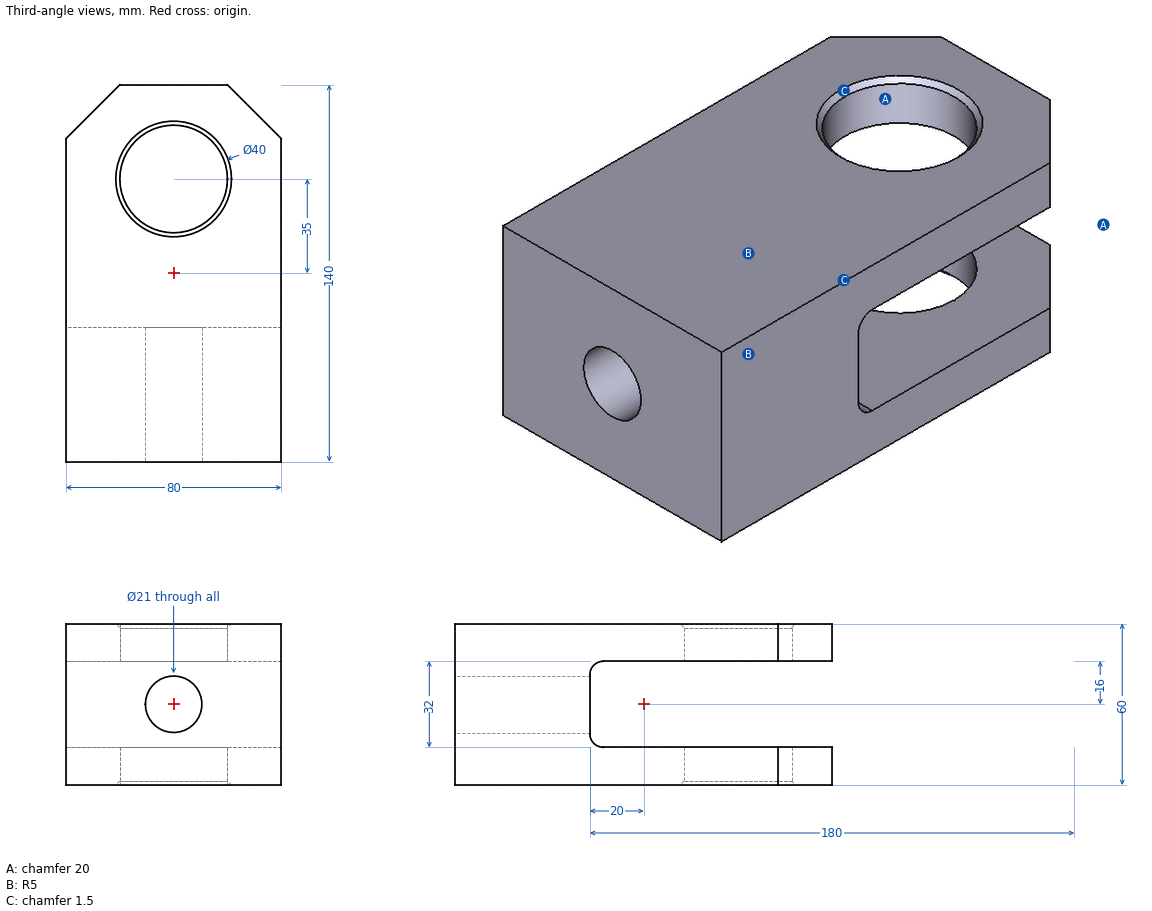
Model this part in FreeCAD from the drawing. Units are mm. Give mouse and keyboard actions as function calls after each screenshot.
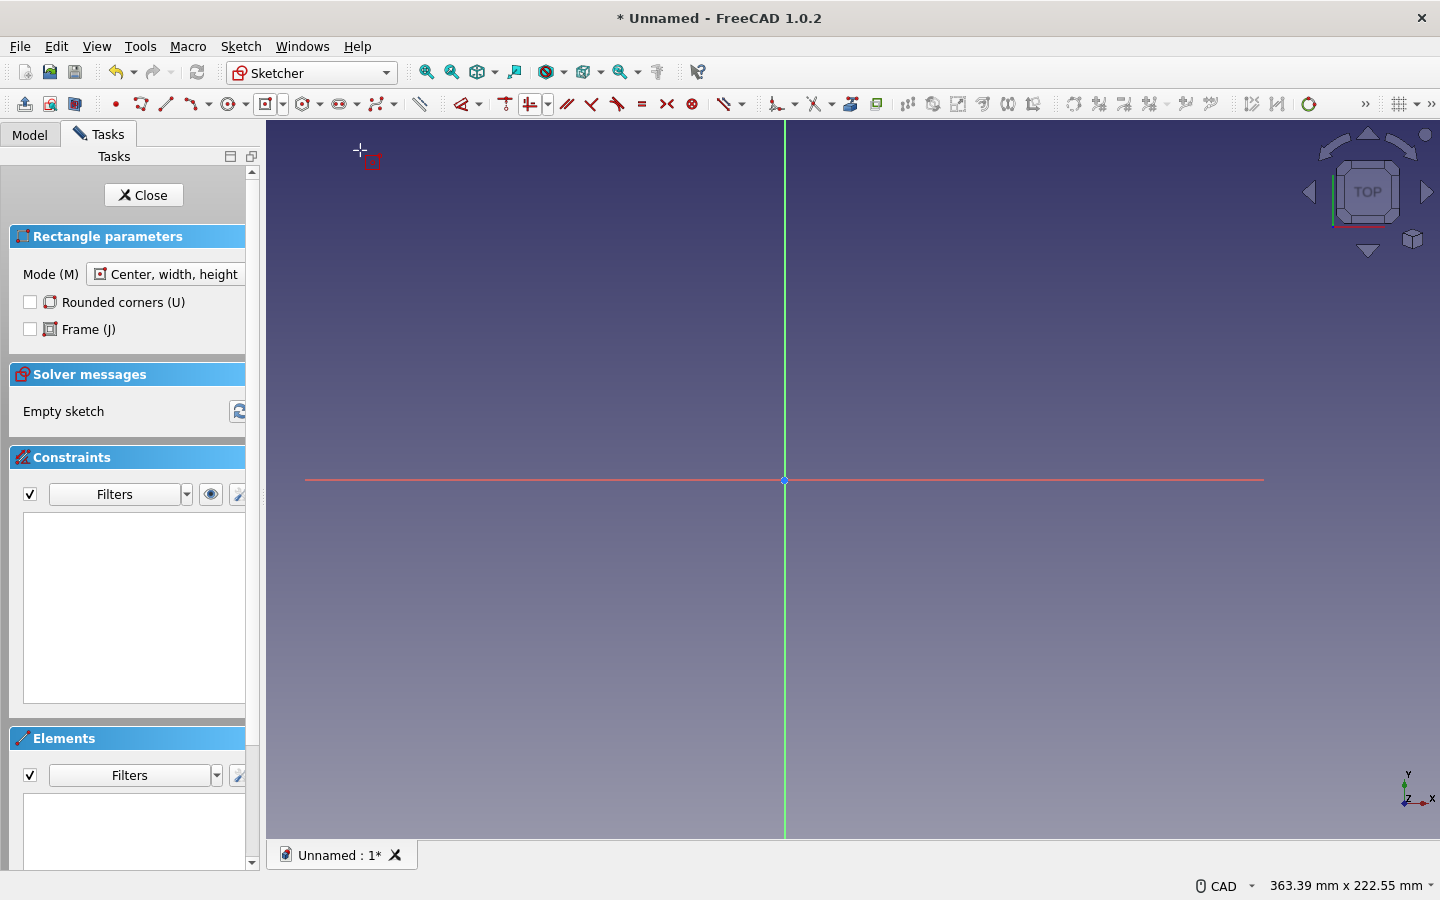
click(785, 480)
move(914, 254)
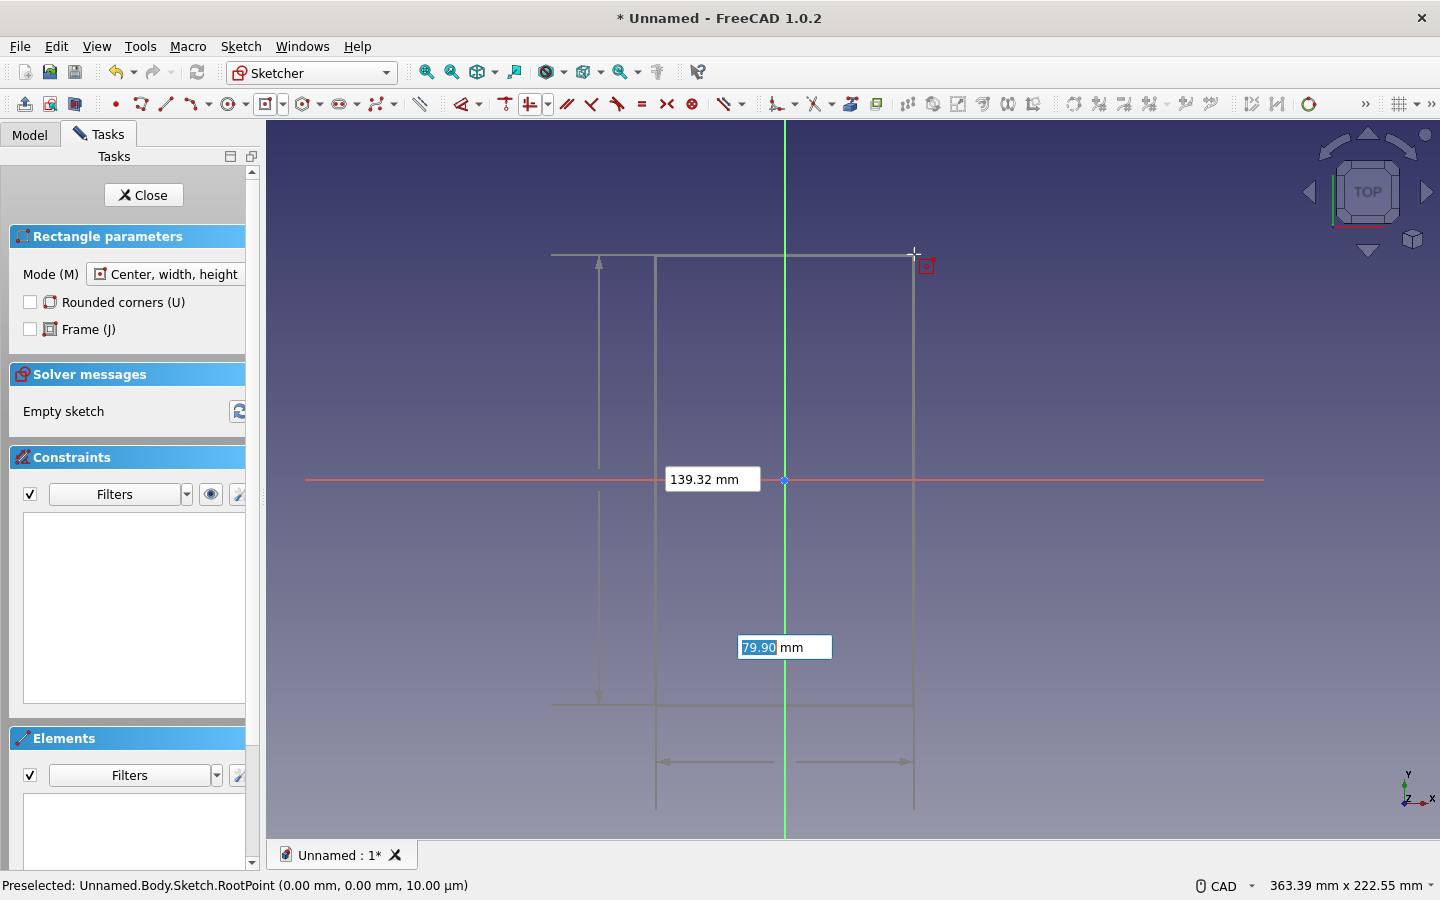
text(80)
key(Tab)
text(140)
key(Return)
key(Escape)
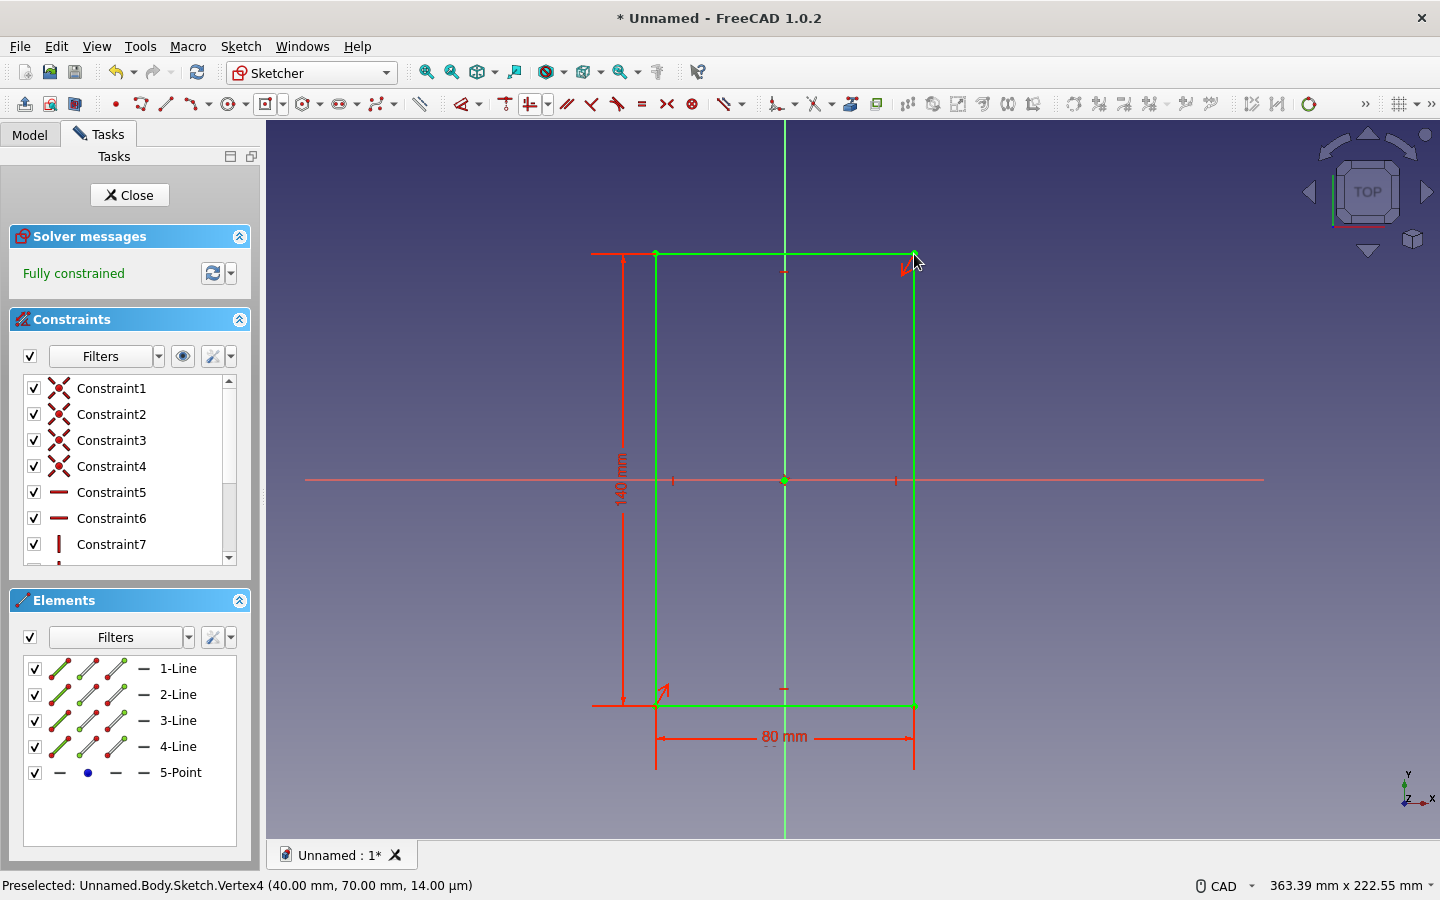
click(130, 195)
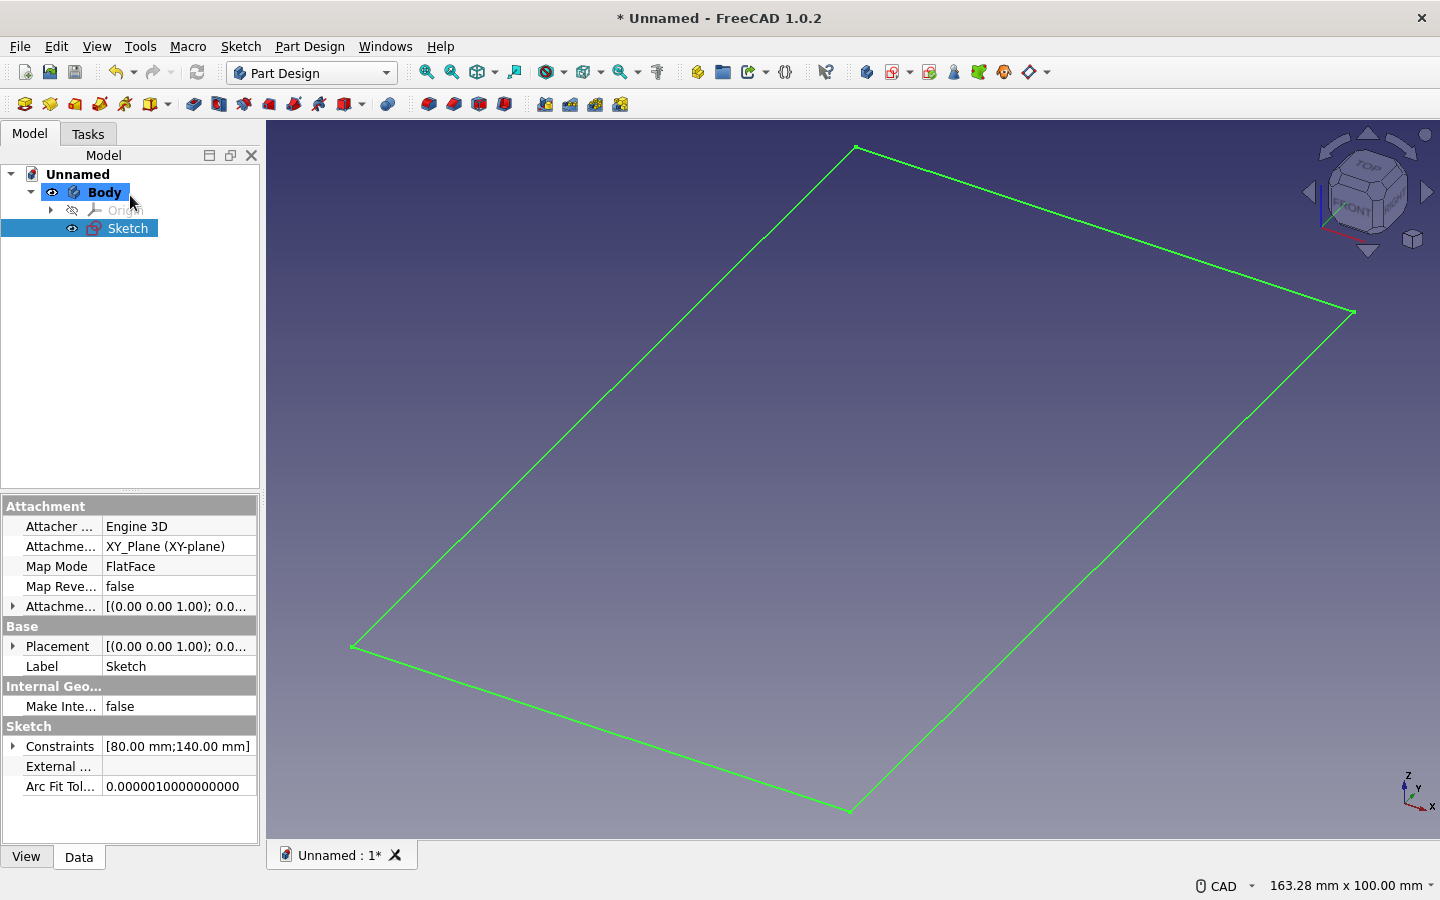
click(25, 104)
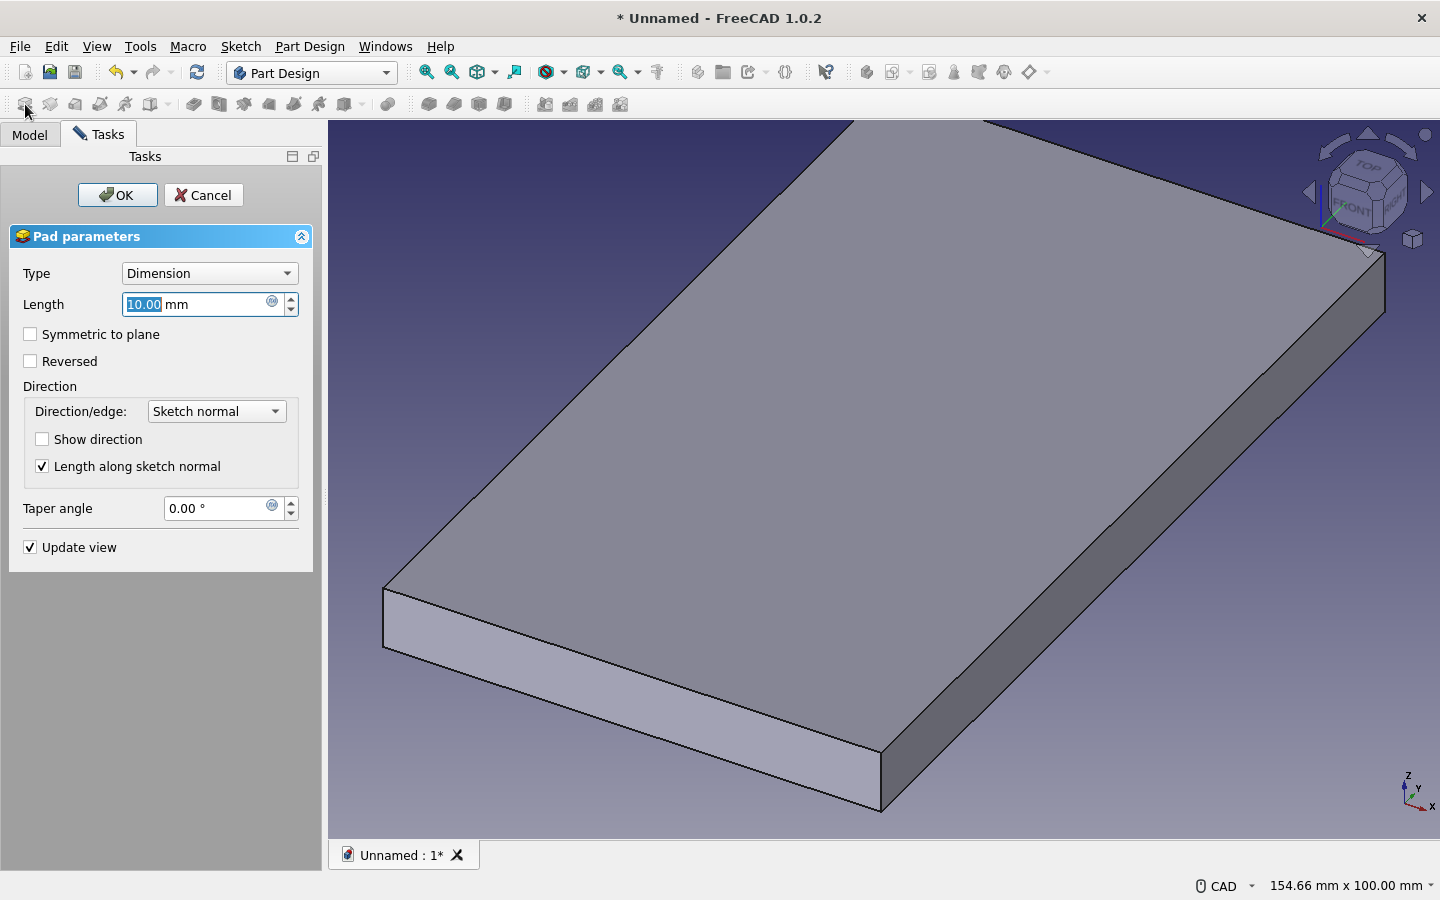
text(60)
key(Tab)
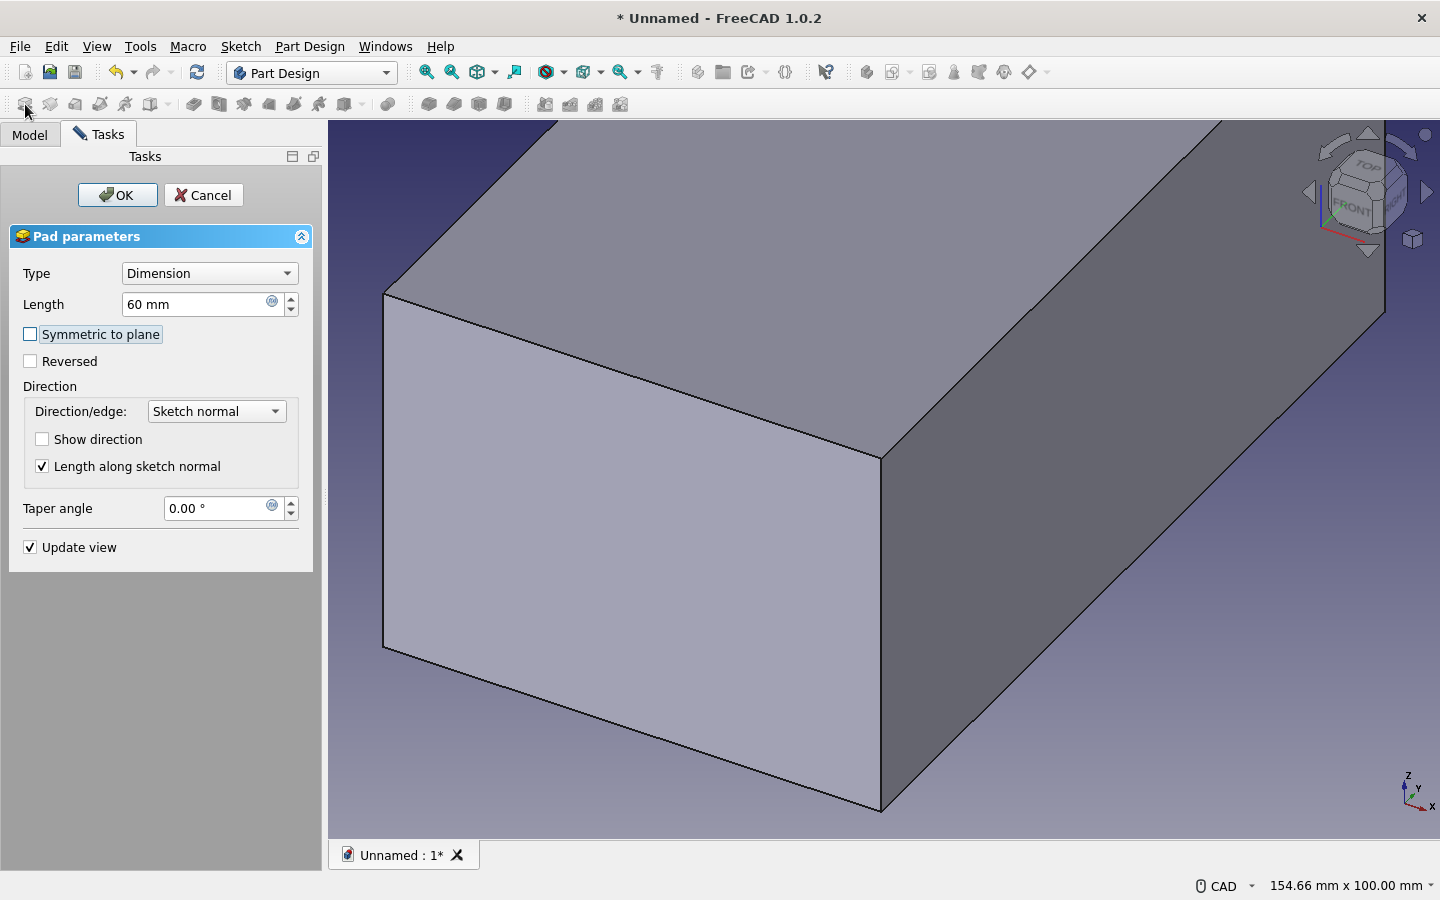
click(31, 334)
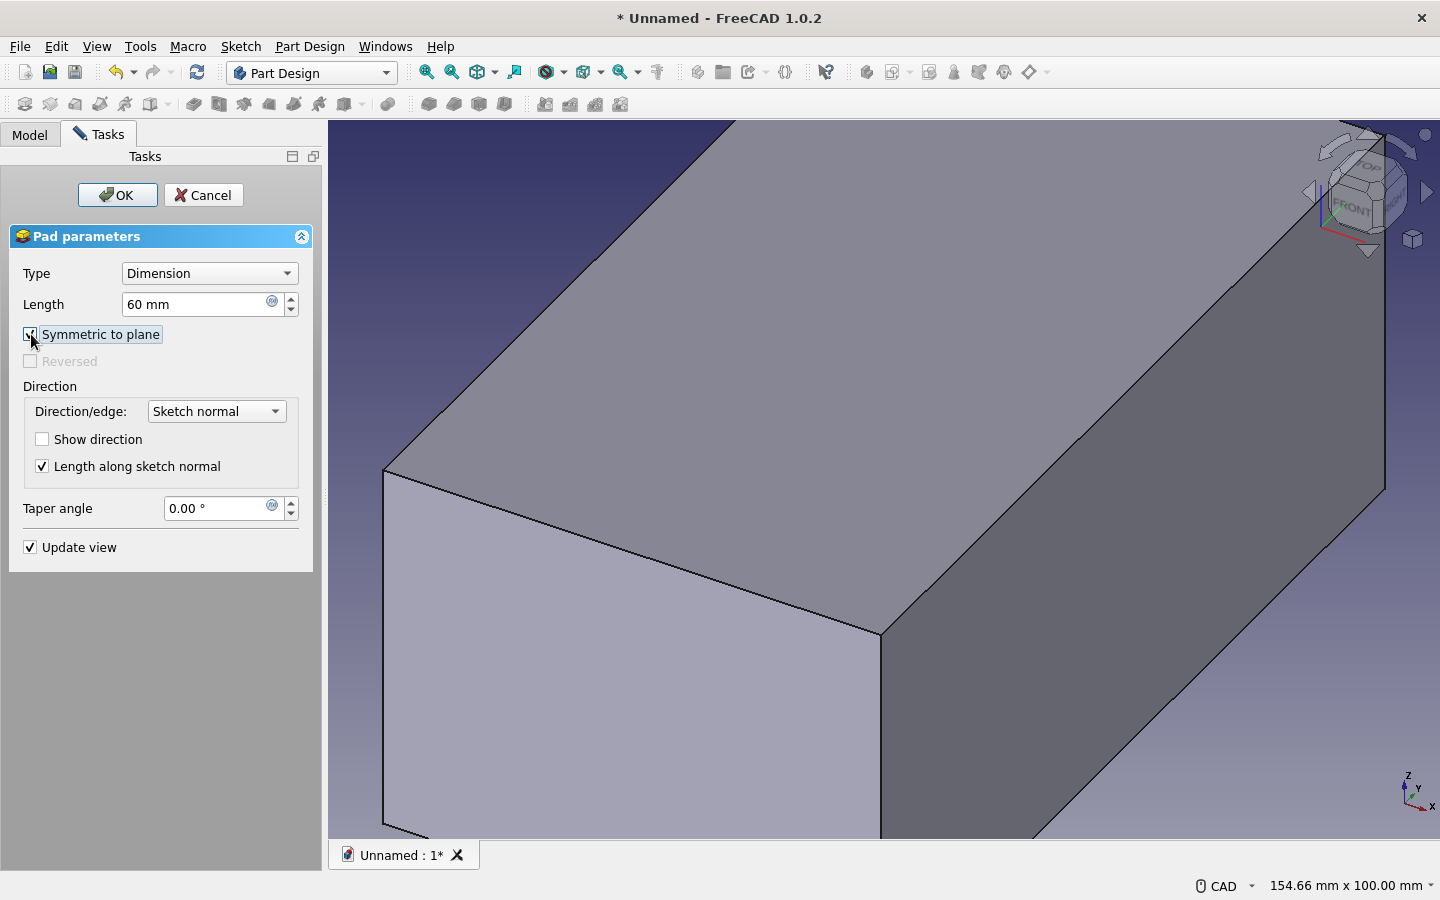
click(118, 195)